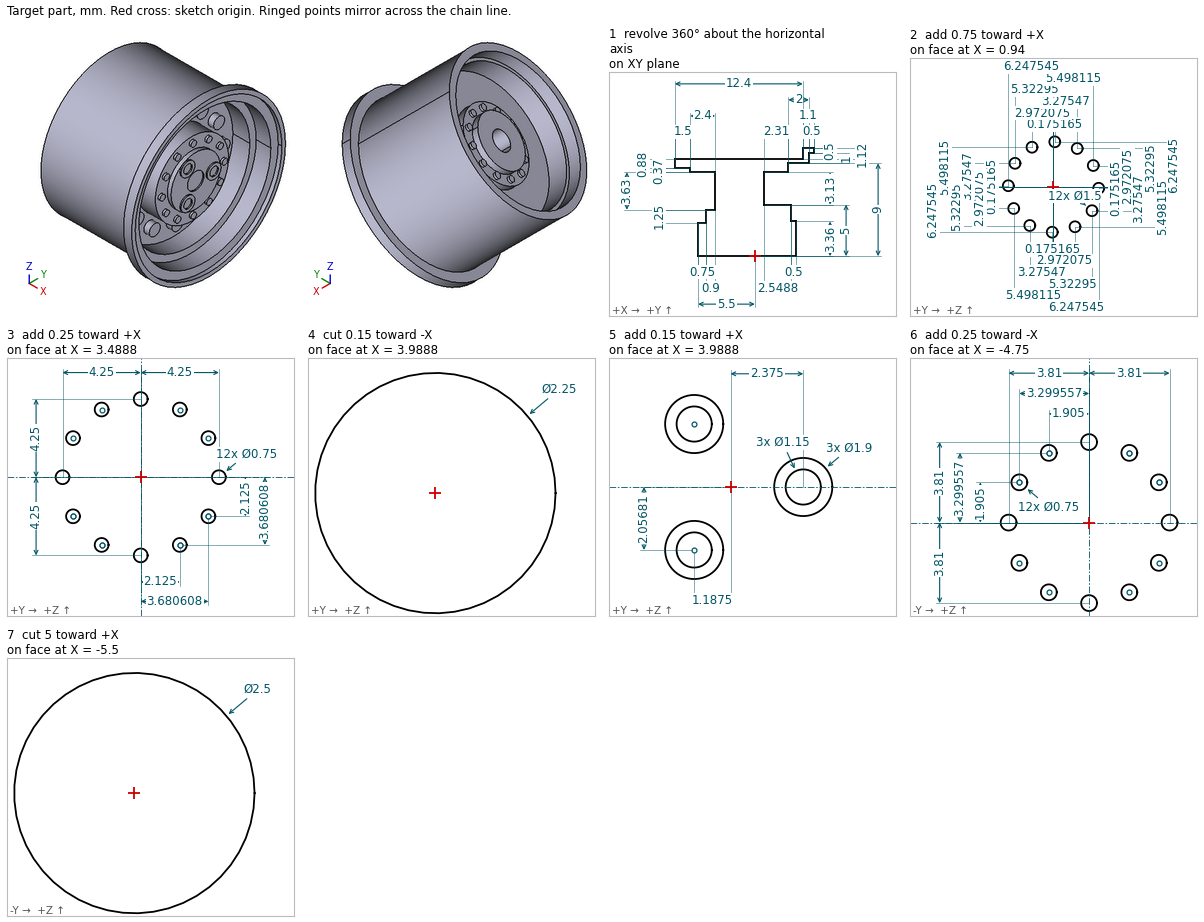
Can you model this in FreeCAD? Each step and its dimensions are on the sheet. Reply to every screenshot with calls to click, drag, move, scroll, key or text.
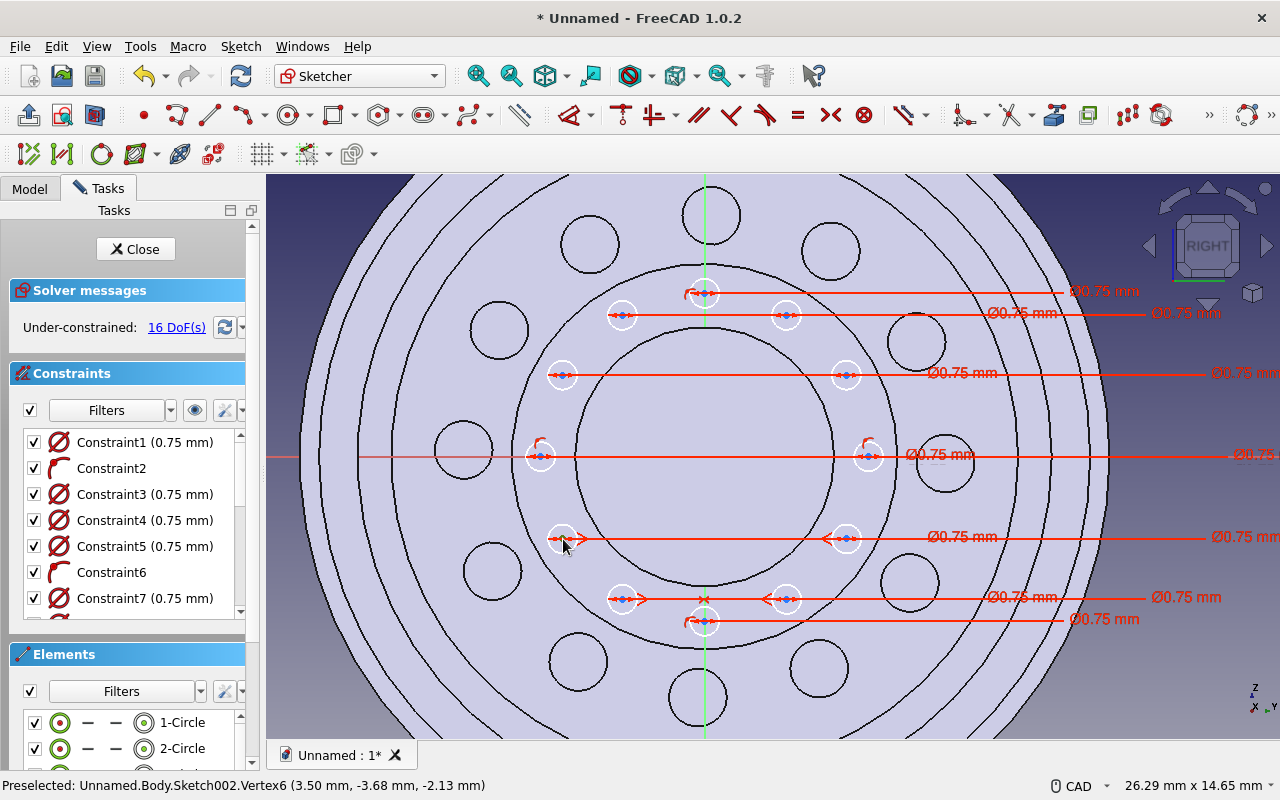
click(563, 375)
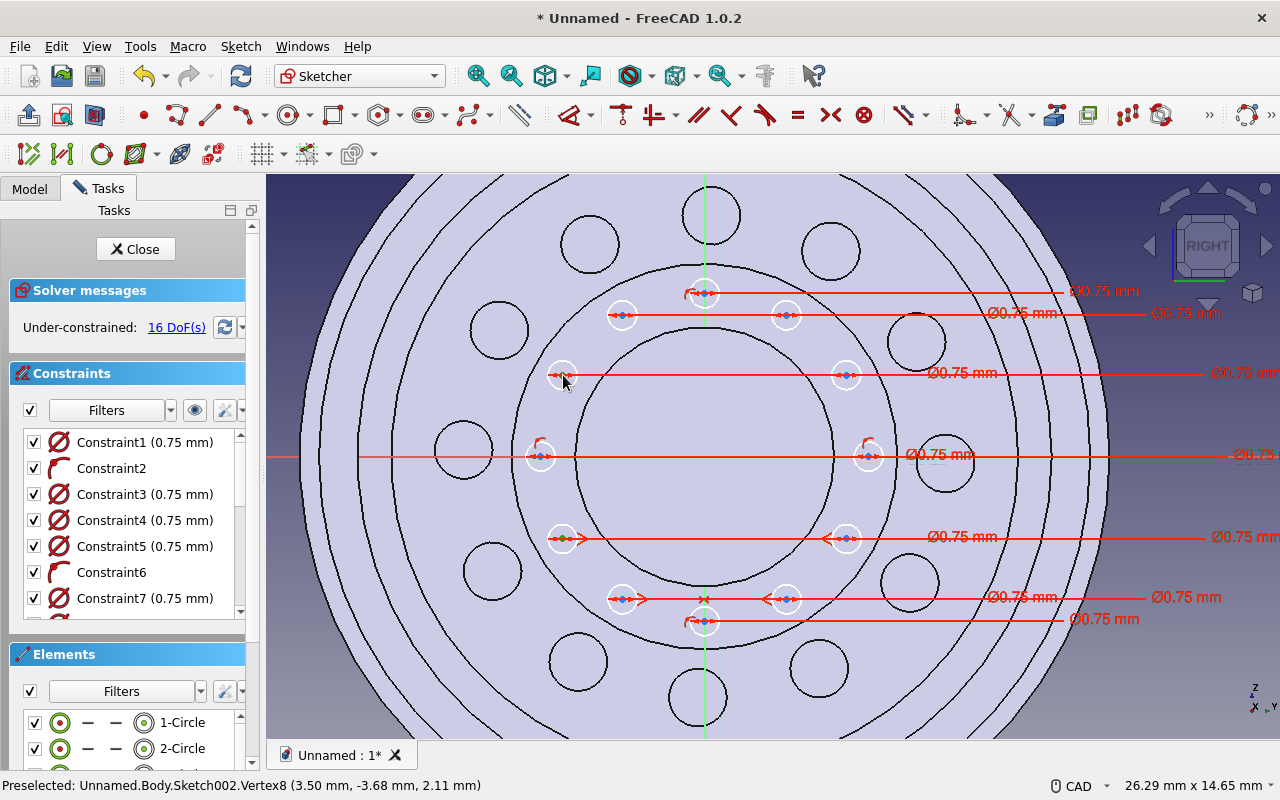
click(353, 457)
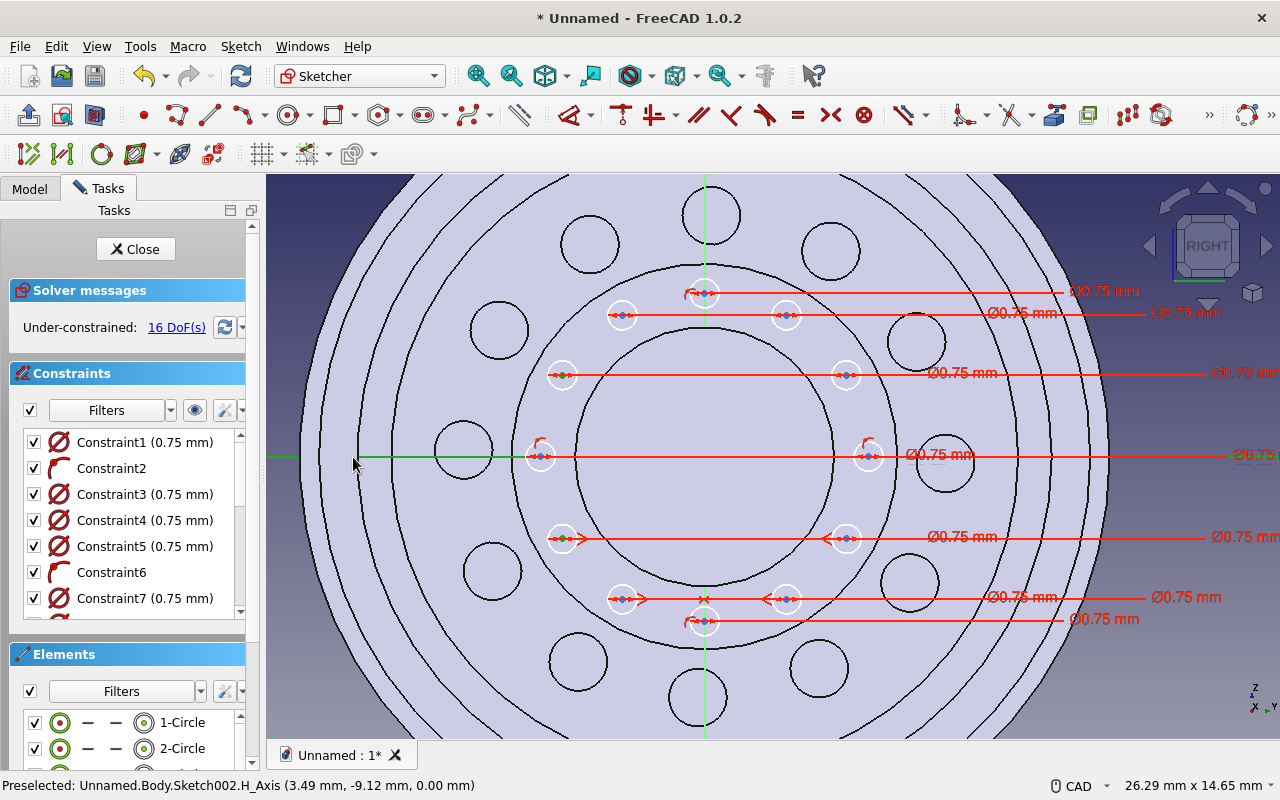
click(831, 116)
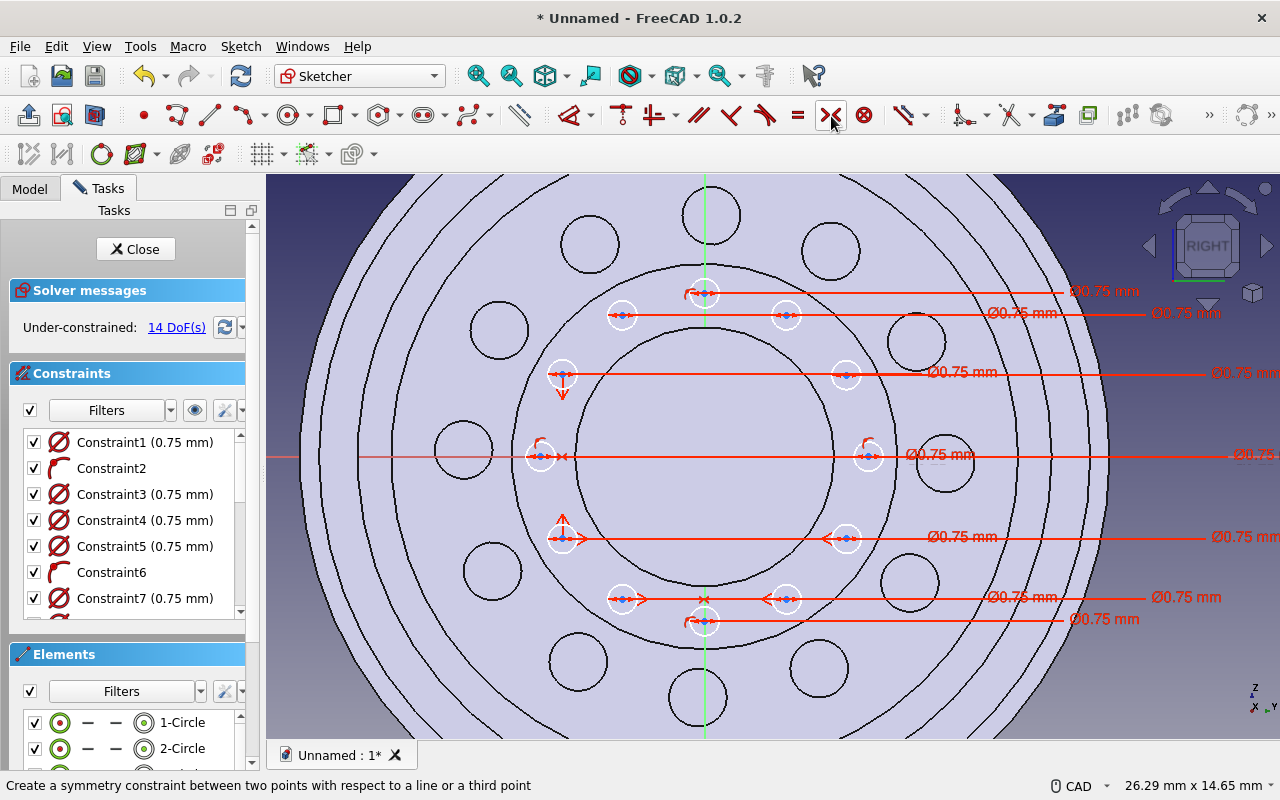
click(623, 599)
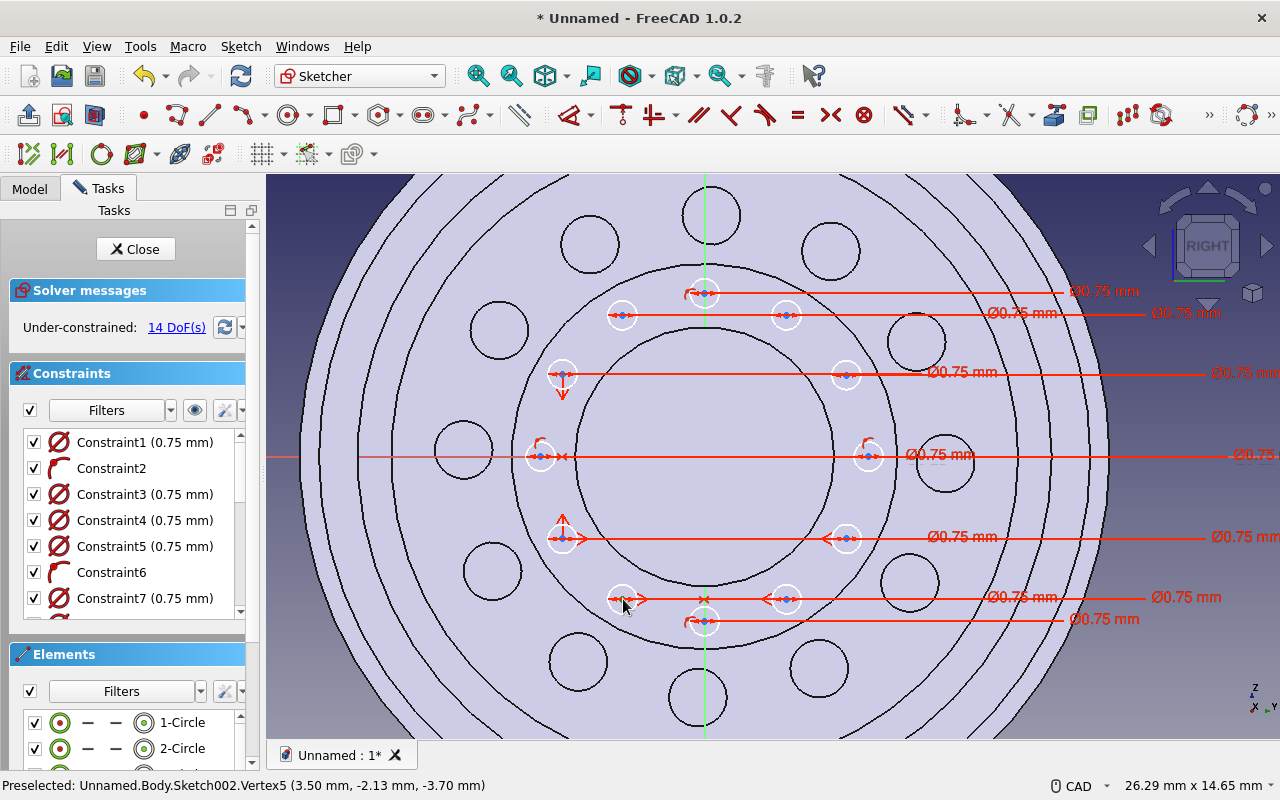
click(622, 315)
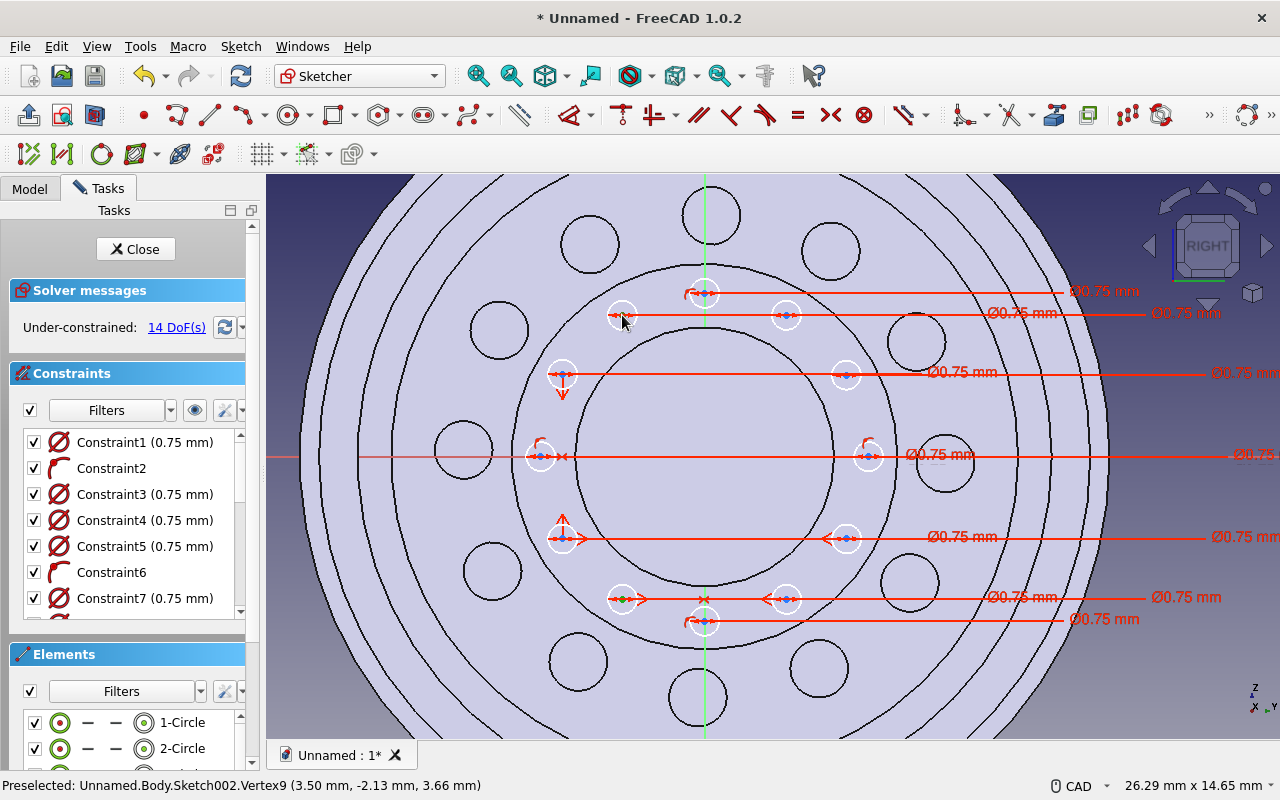
click(353, 457)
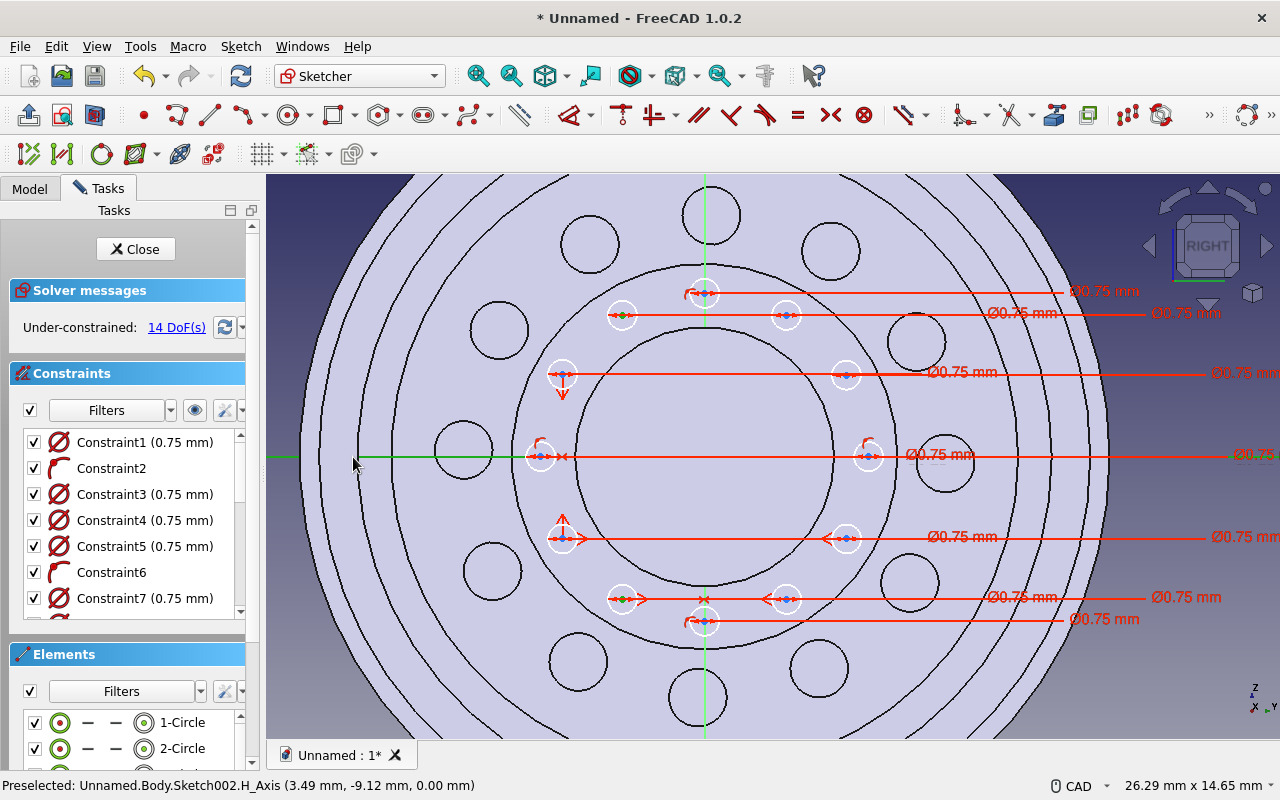
click(831, 116)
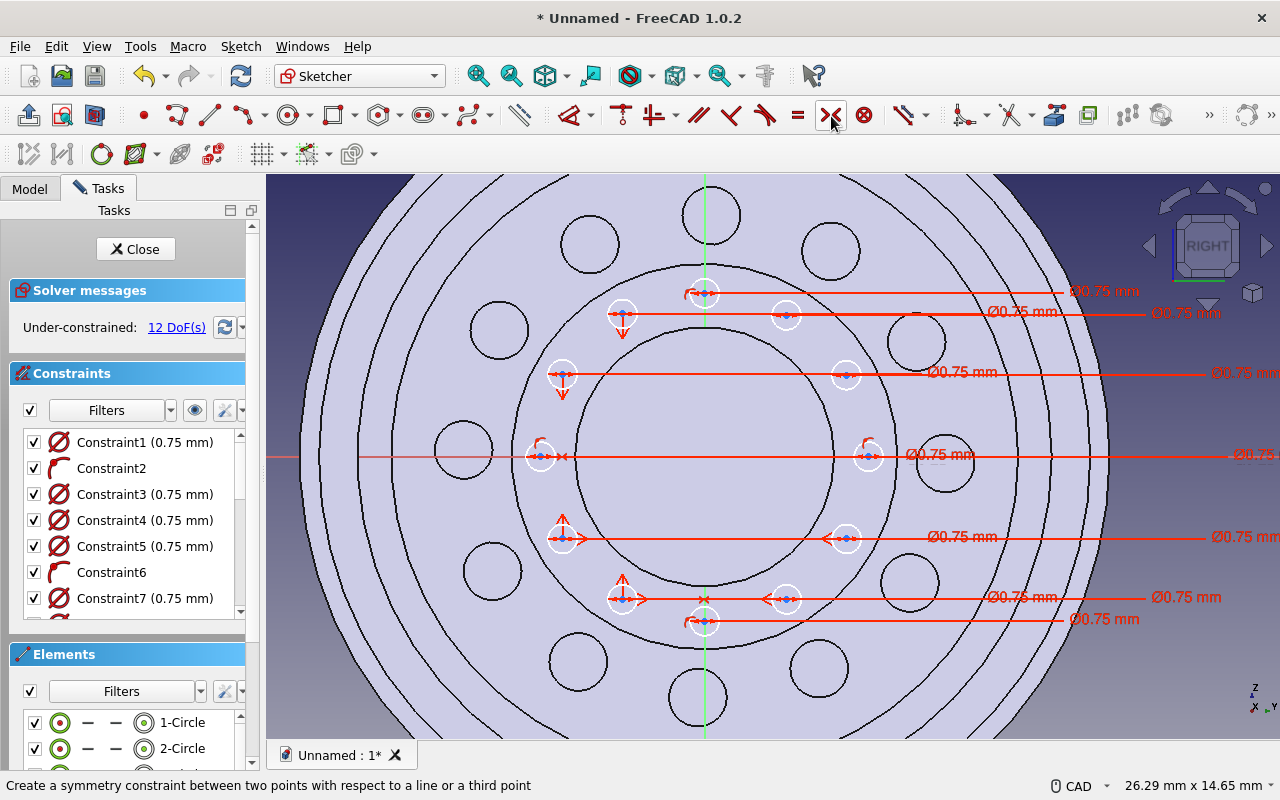
click(787, 599)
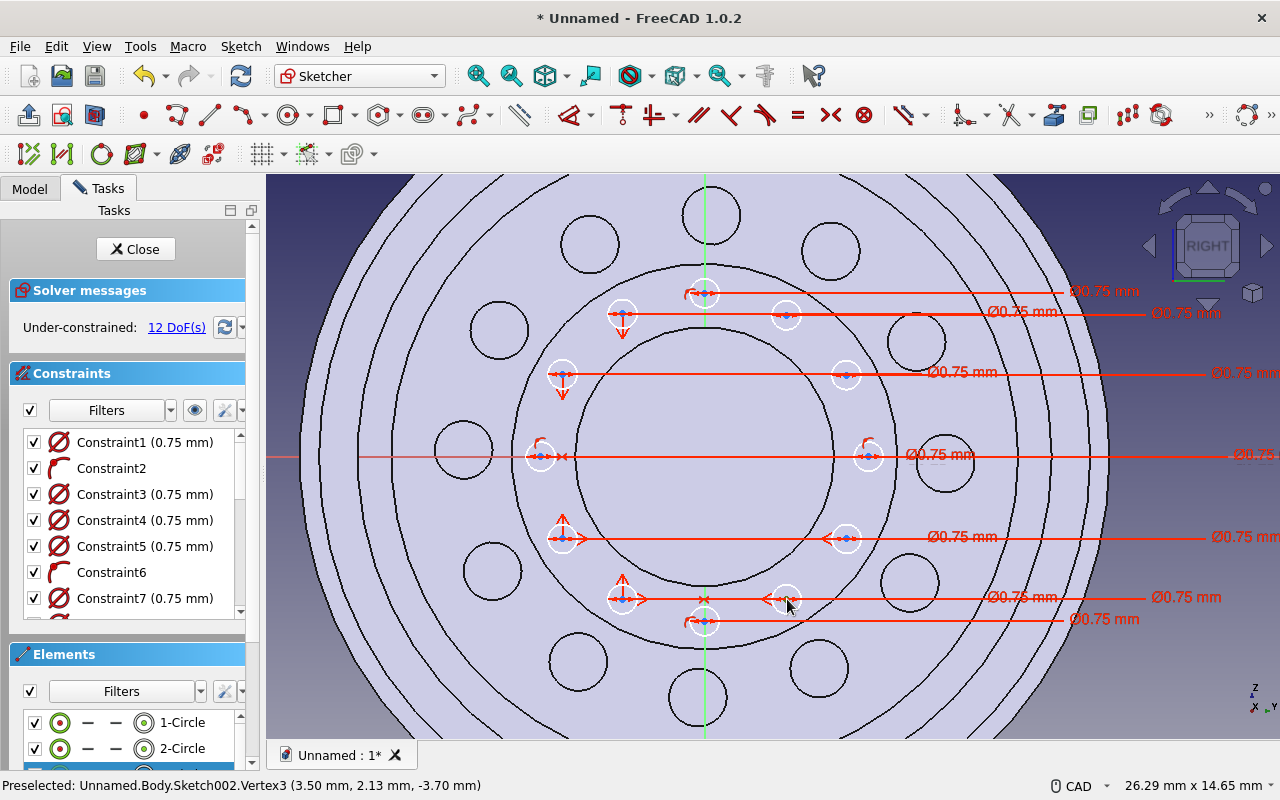
click(786, 315)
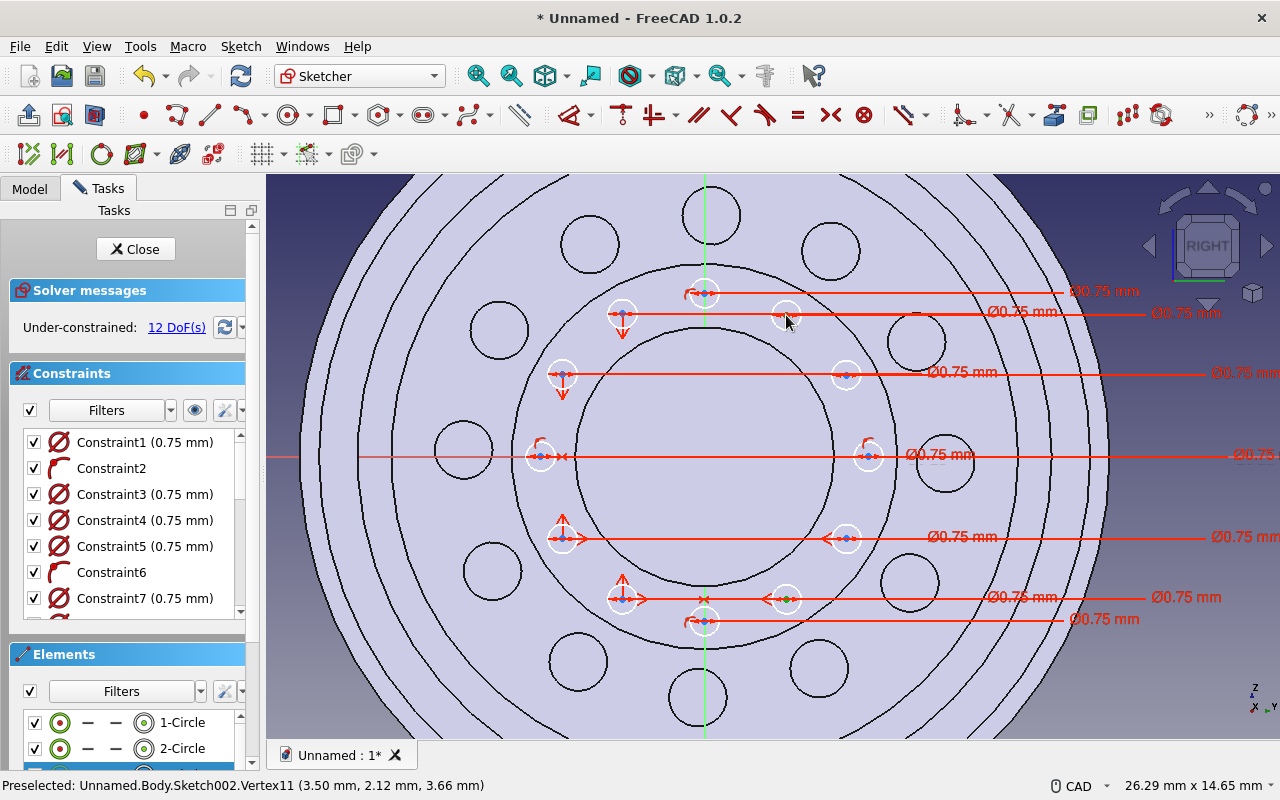
click(353, 457)